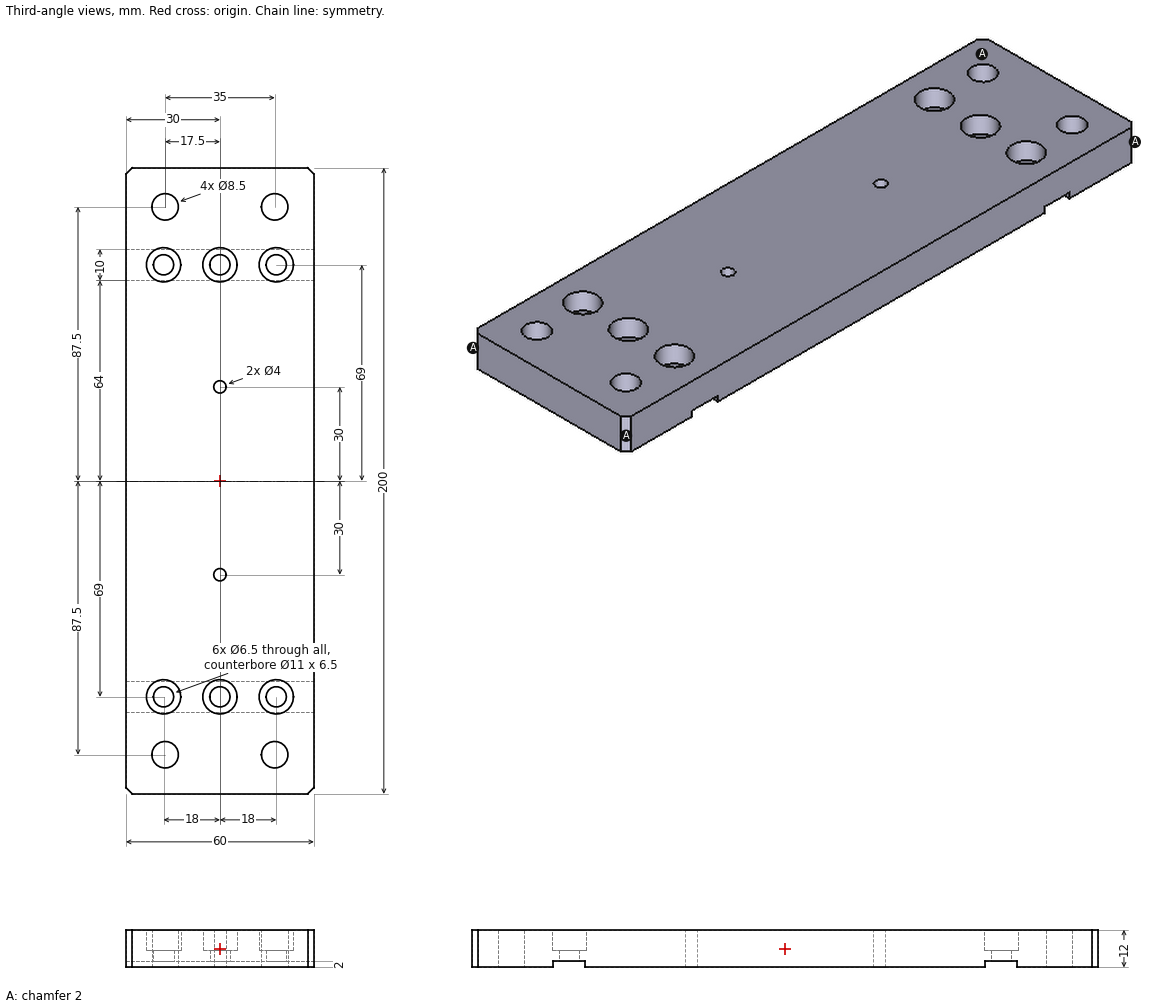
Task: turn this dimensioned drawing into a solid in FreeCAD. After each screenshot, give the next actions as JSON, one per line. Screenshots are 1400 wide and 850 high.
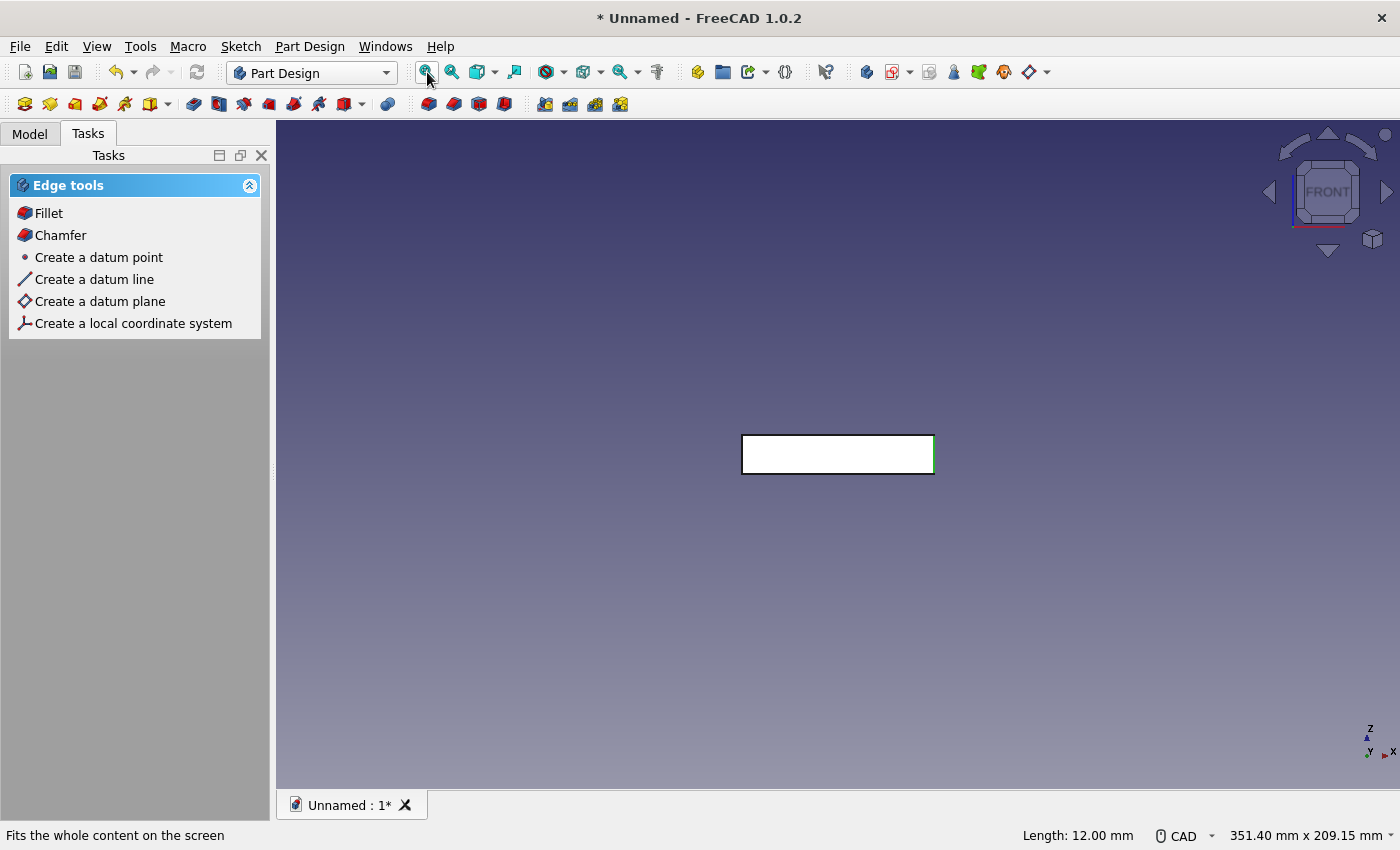
{"action": "left_click", "coordinate": [742, 454], "text": "ctrl"}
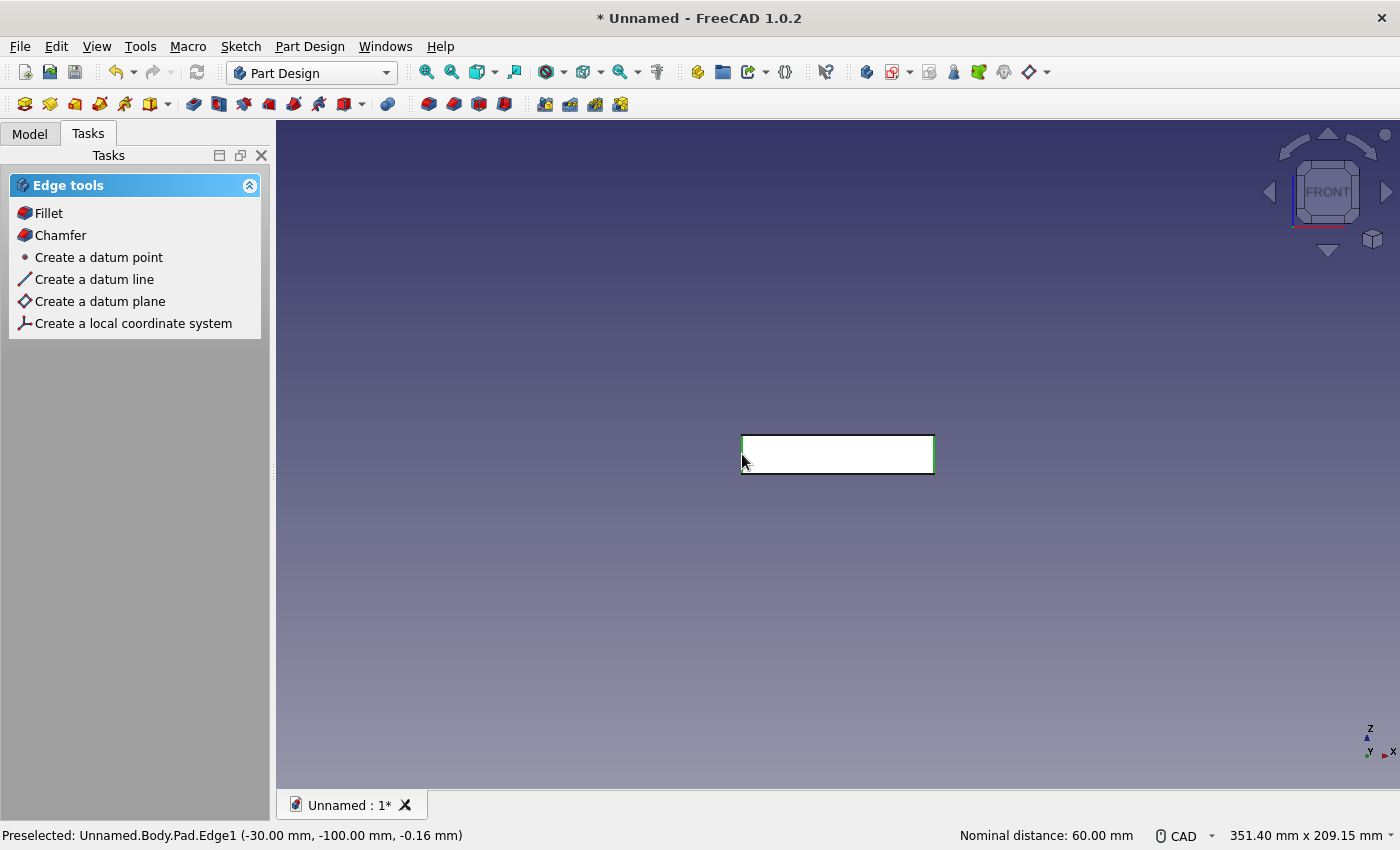
{"action": "key", "text": "3"}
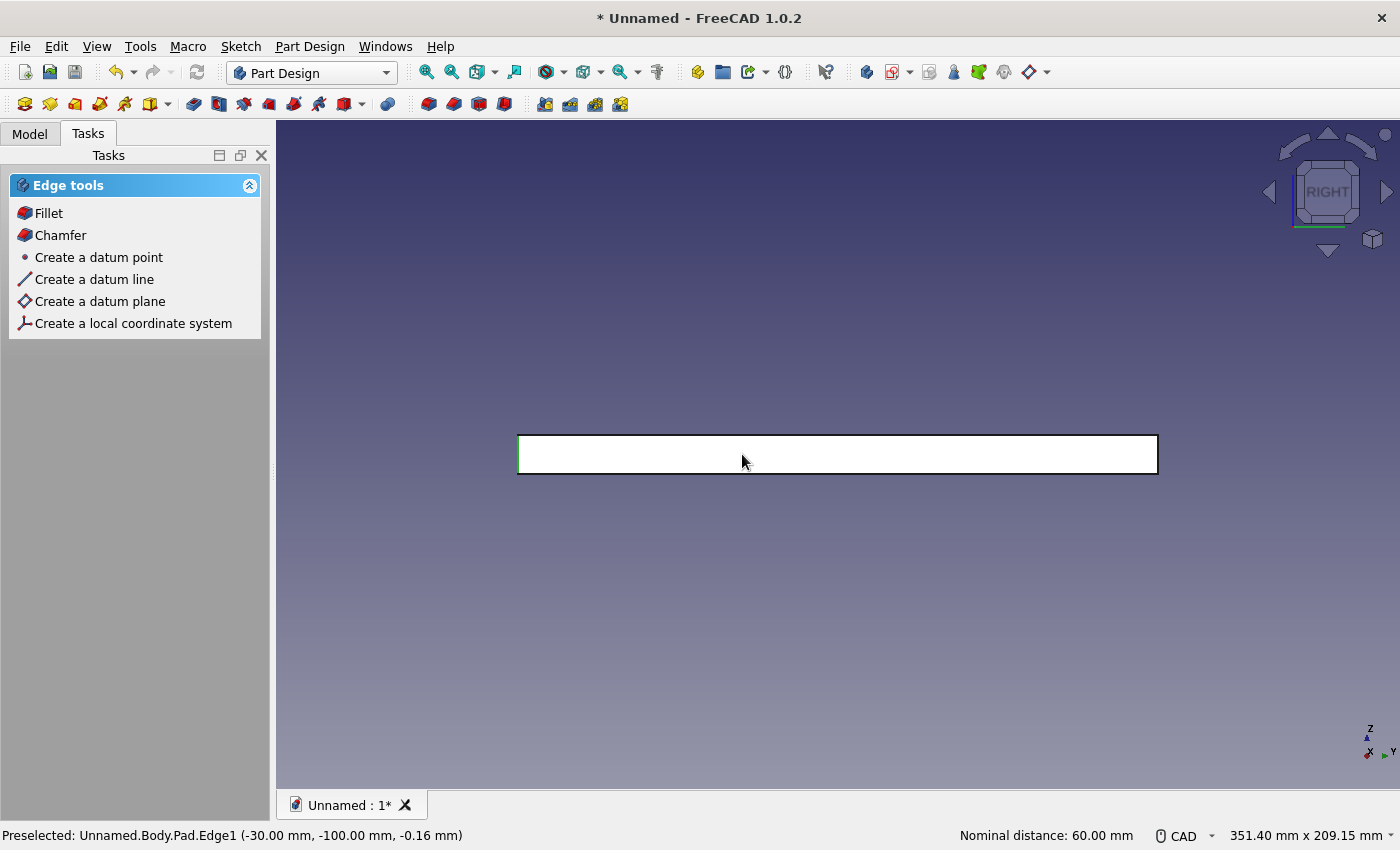
{"action": "left_click", "coordinate": [1158, 453], "text": "ctrl"}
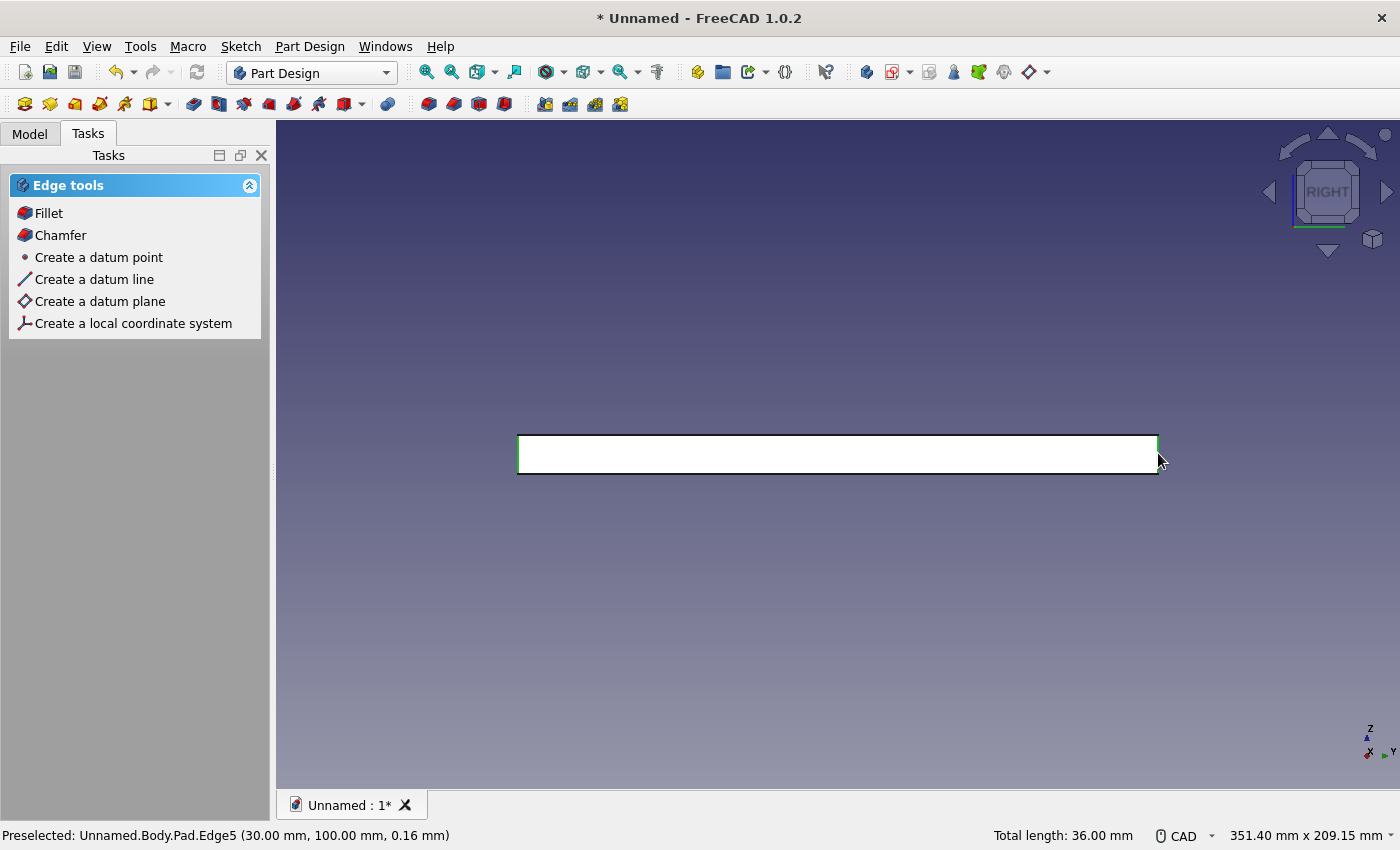
{"action": "key", "text": "5"}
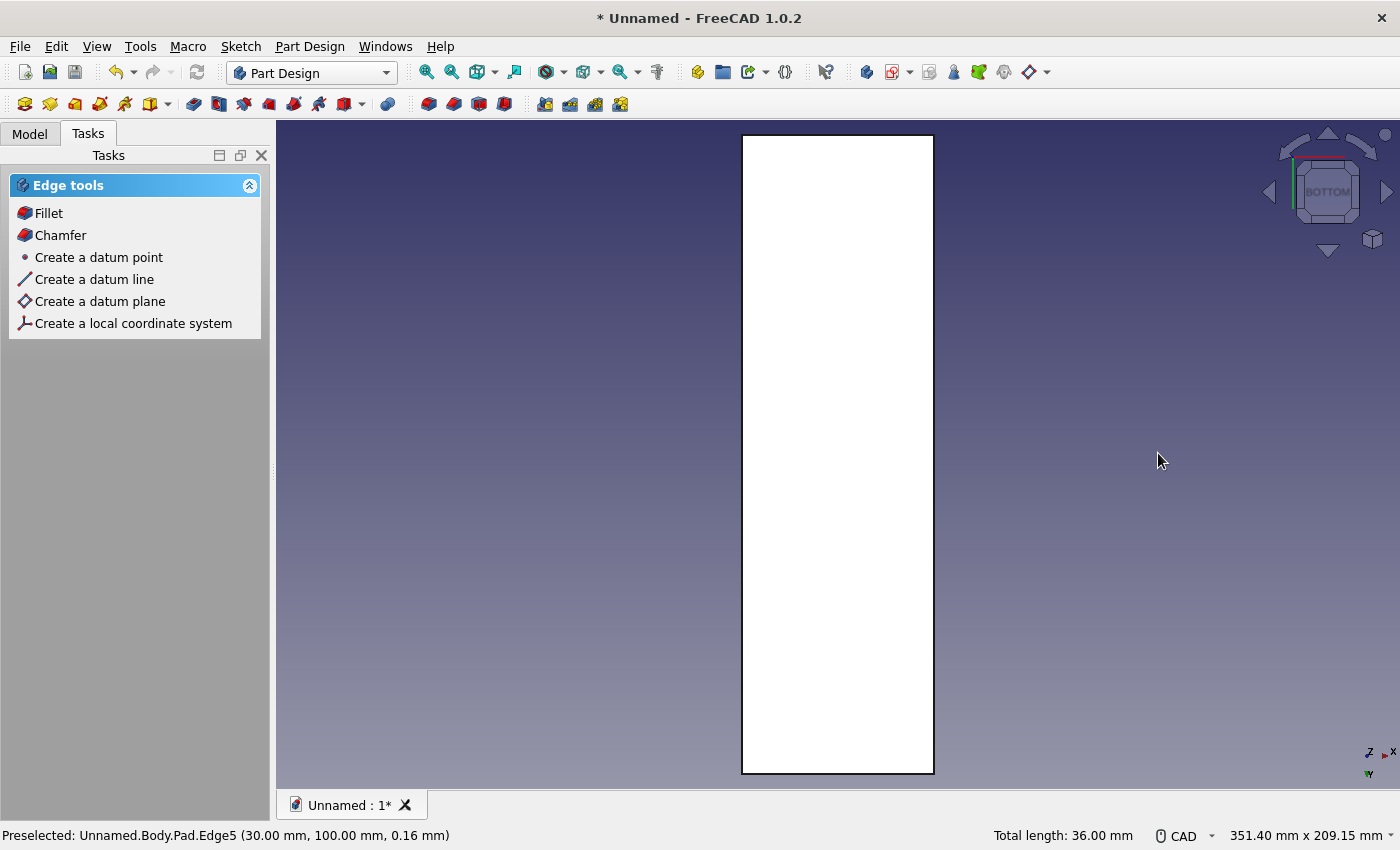
{"action": "key", "text": "4"}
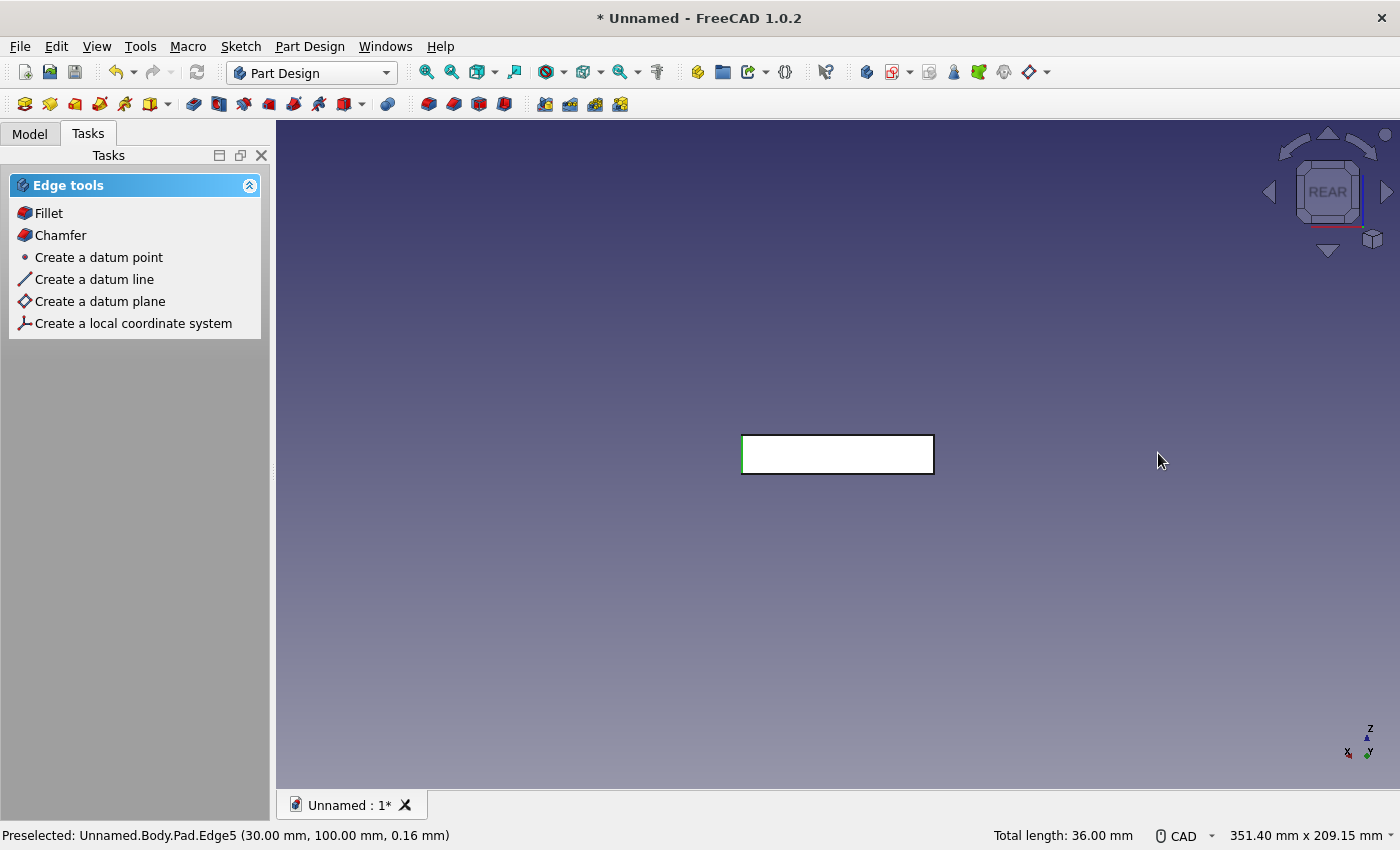
{"action": "left_click", "coordinate": [427, 72]}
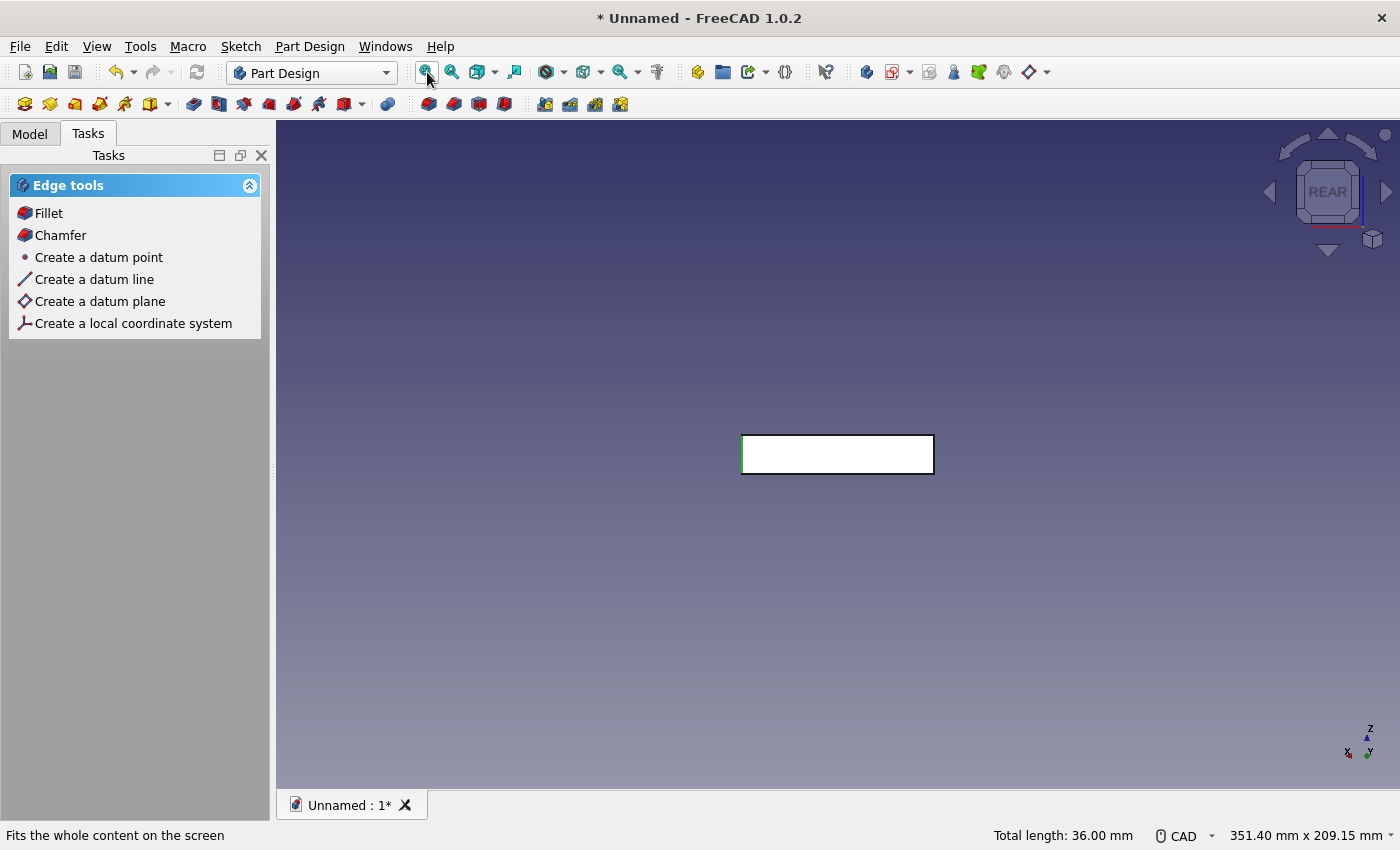
{"action": "left_click", "coordinate": [934, 454], "text": "ctrl"}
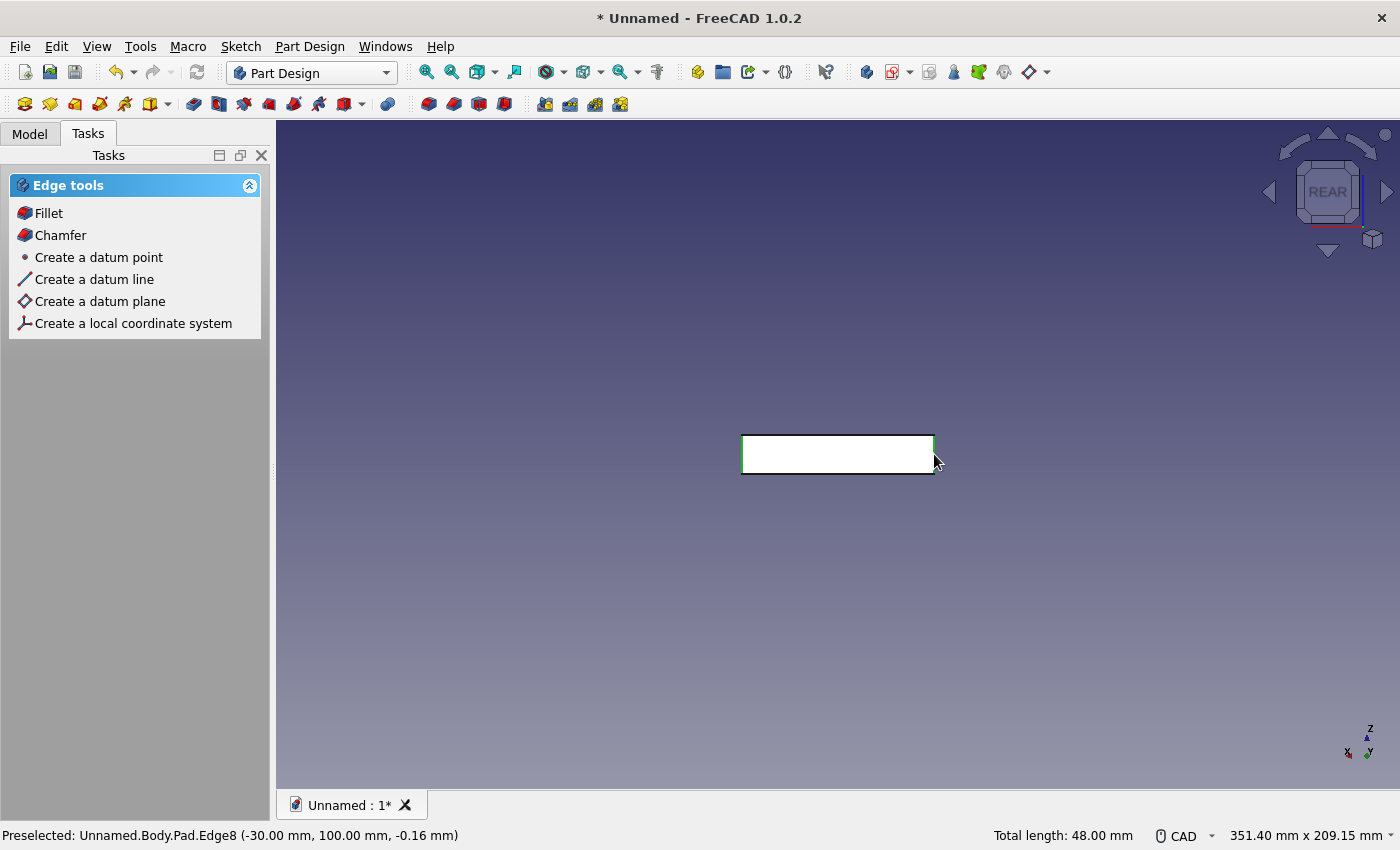
{"action": "left_click", "coordinate": [454, 104]}